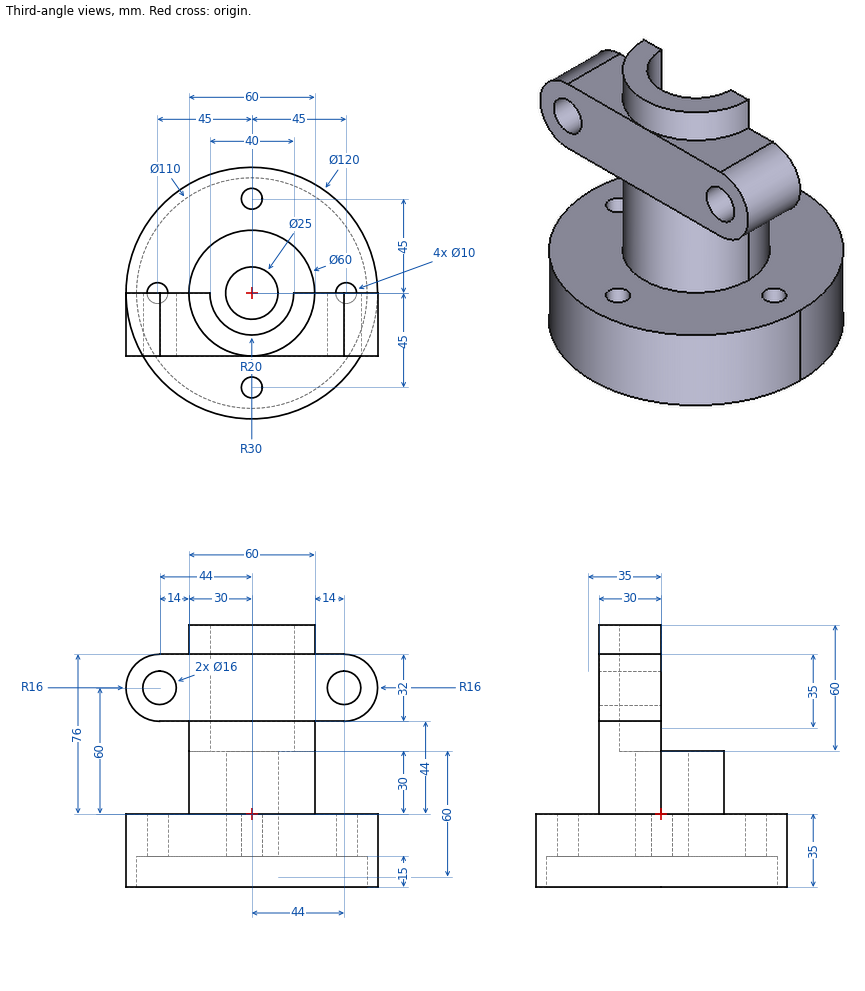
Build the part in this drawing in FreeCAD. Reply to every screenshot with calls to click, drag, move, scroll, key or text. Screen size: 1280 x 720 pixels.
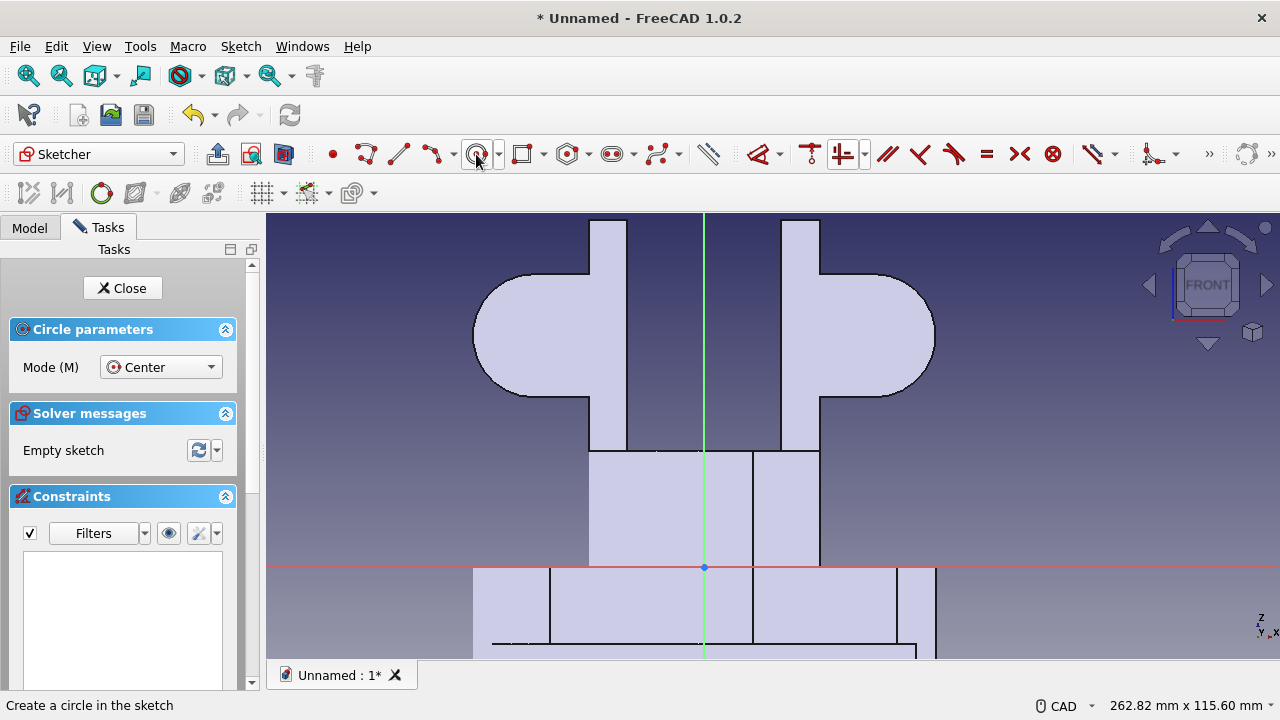
click(535, 336)
move(556, 314)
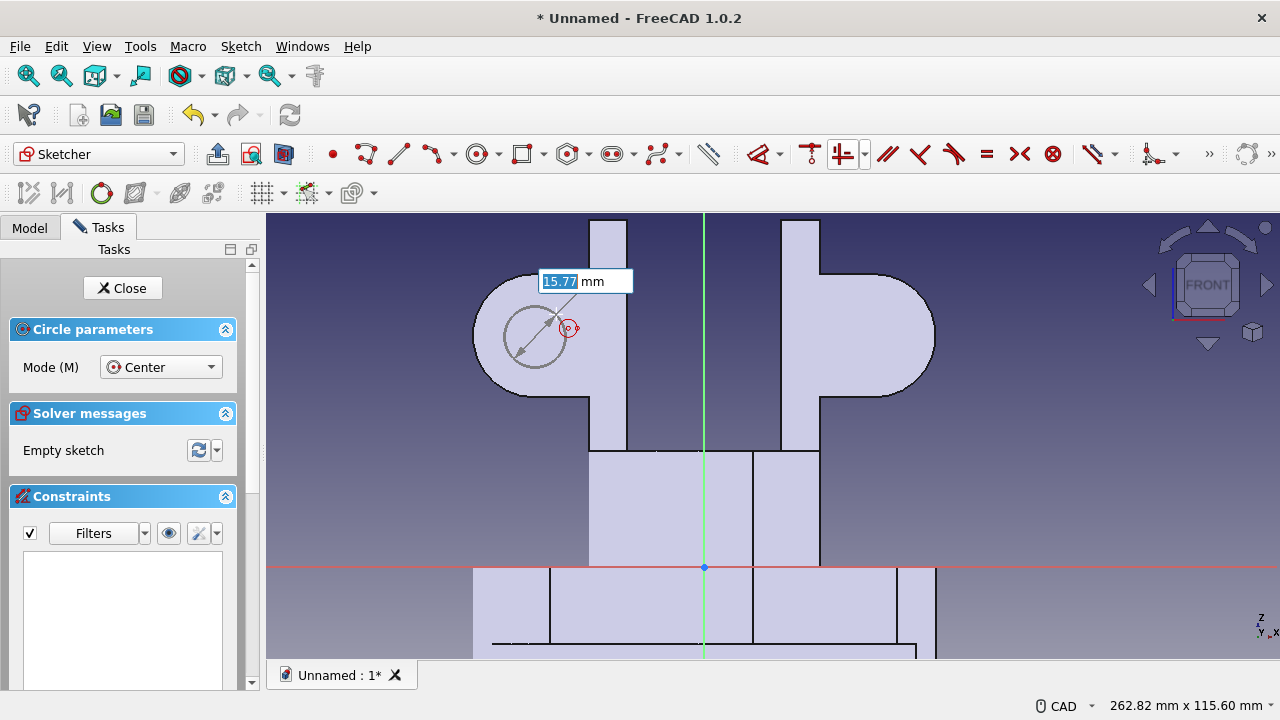
text(16)
key(Return)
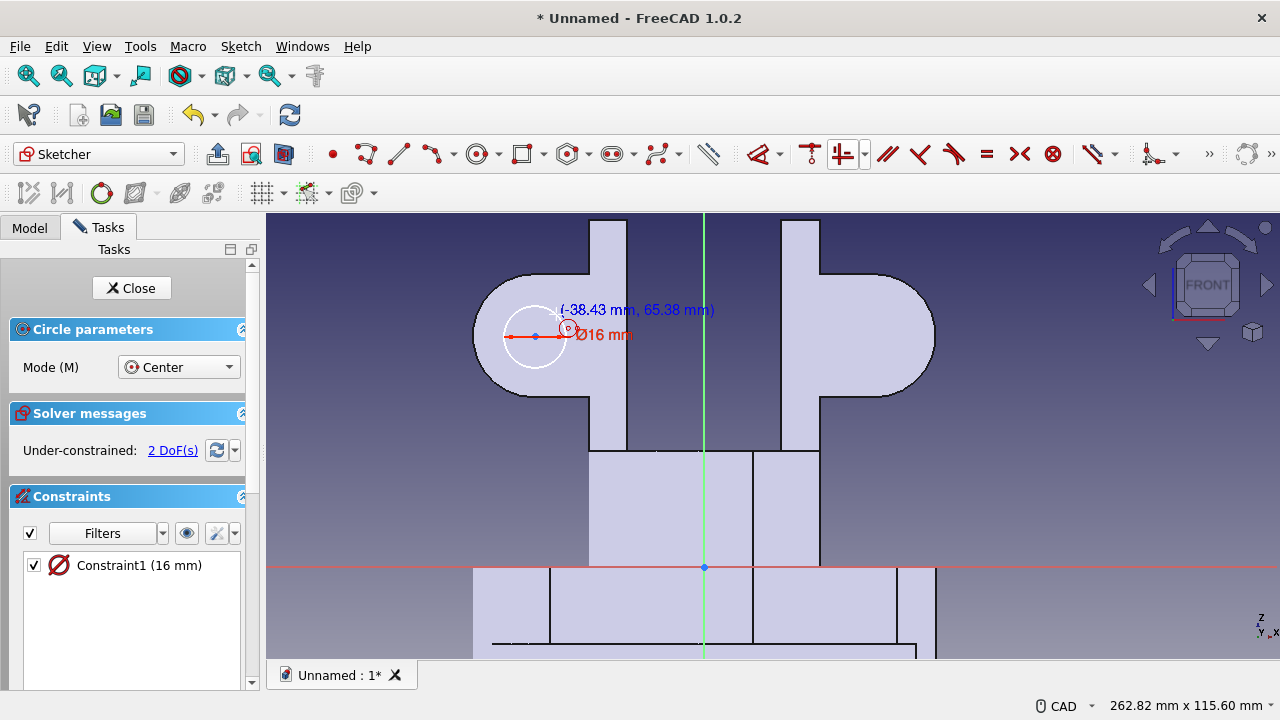
click(874, 336)
move(896, 314)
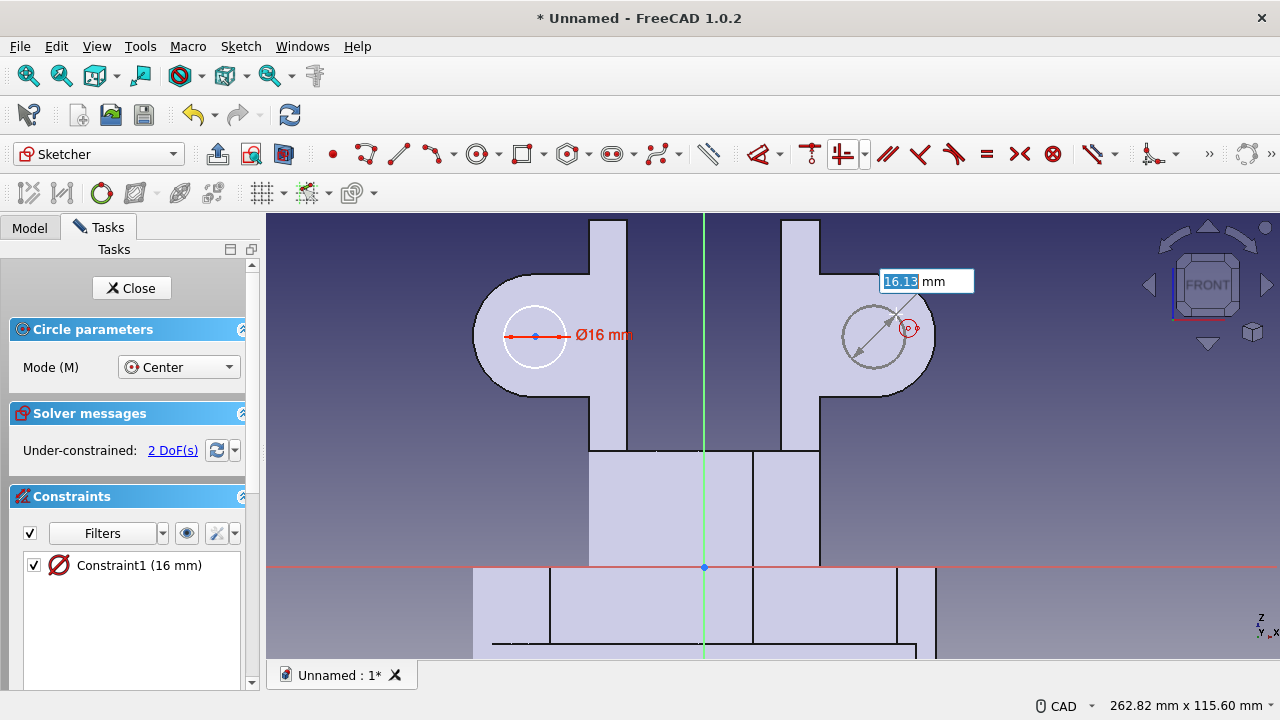
text(16)
key(Return)
key(Escape)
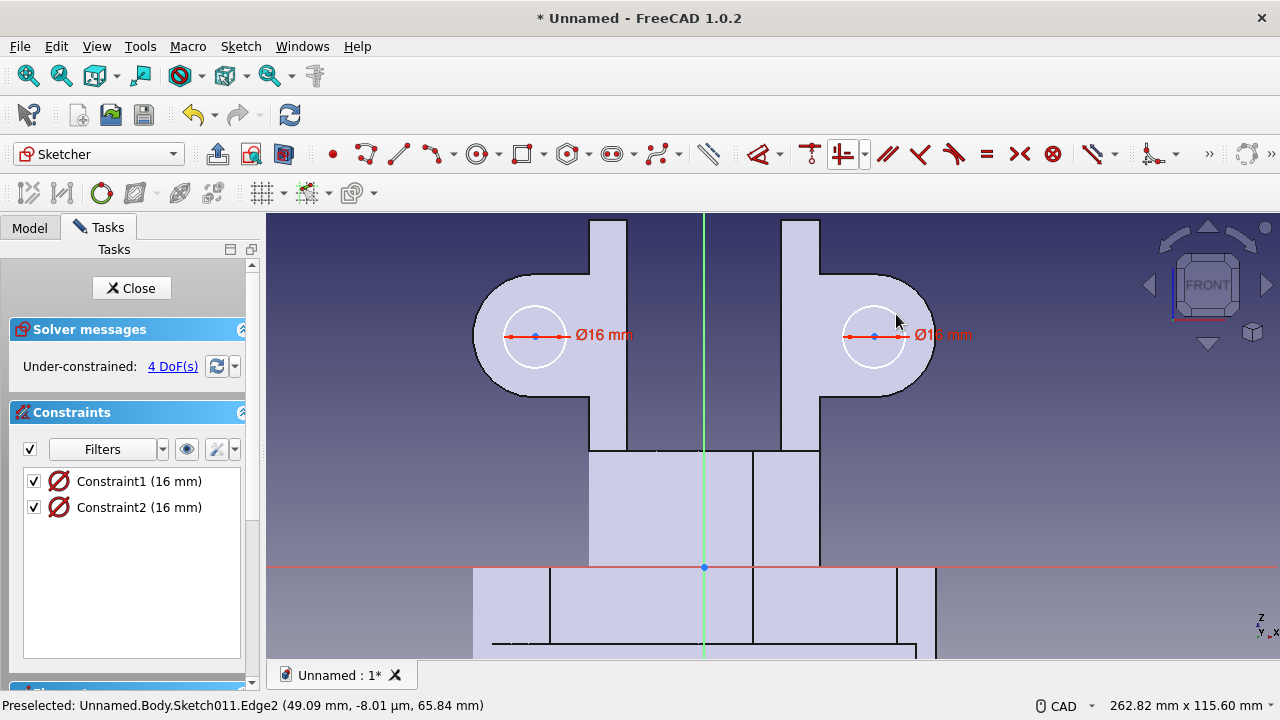
click(535, 337)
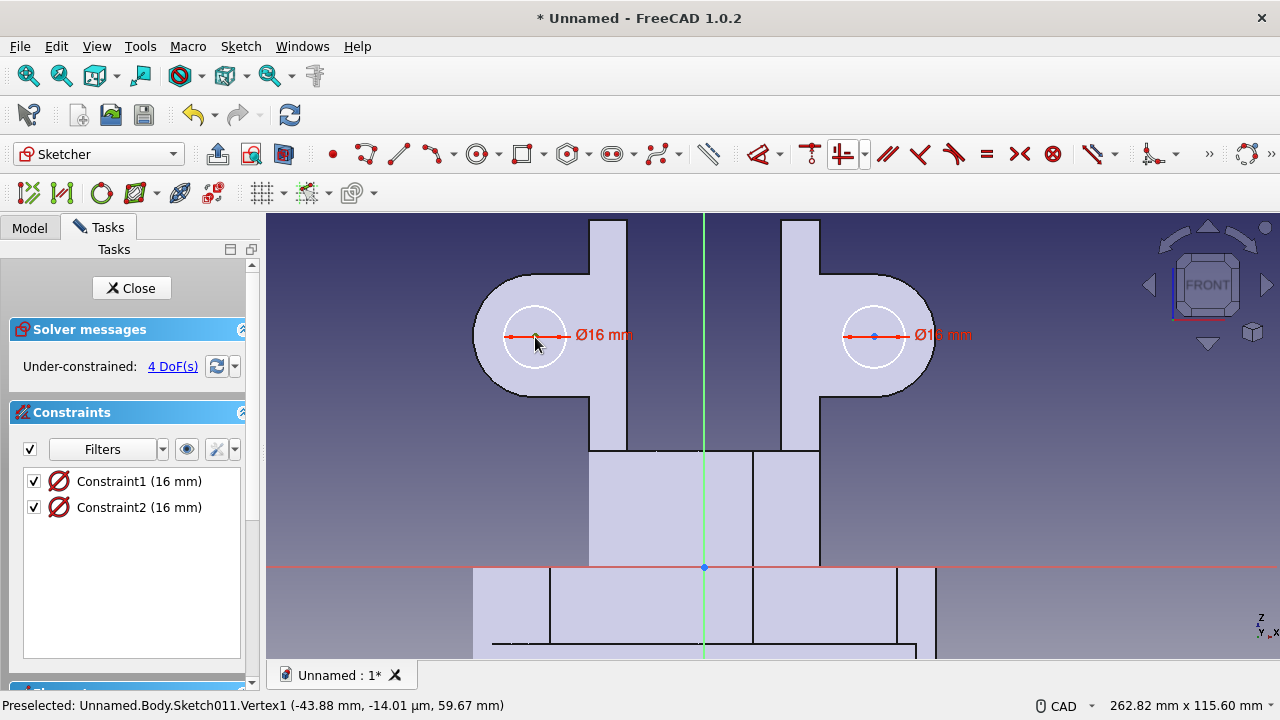
click(874, 337)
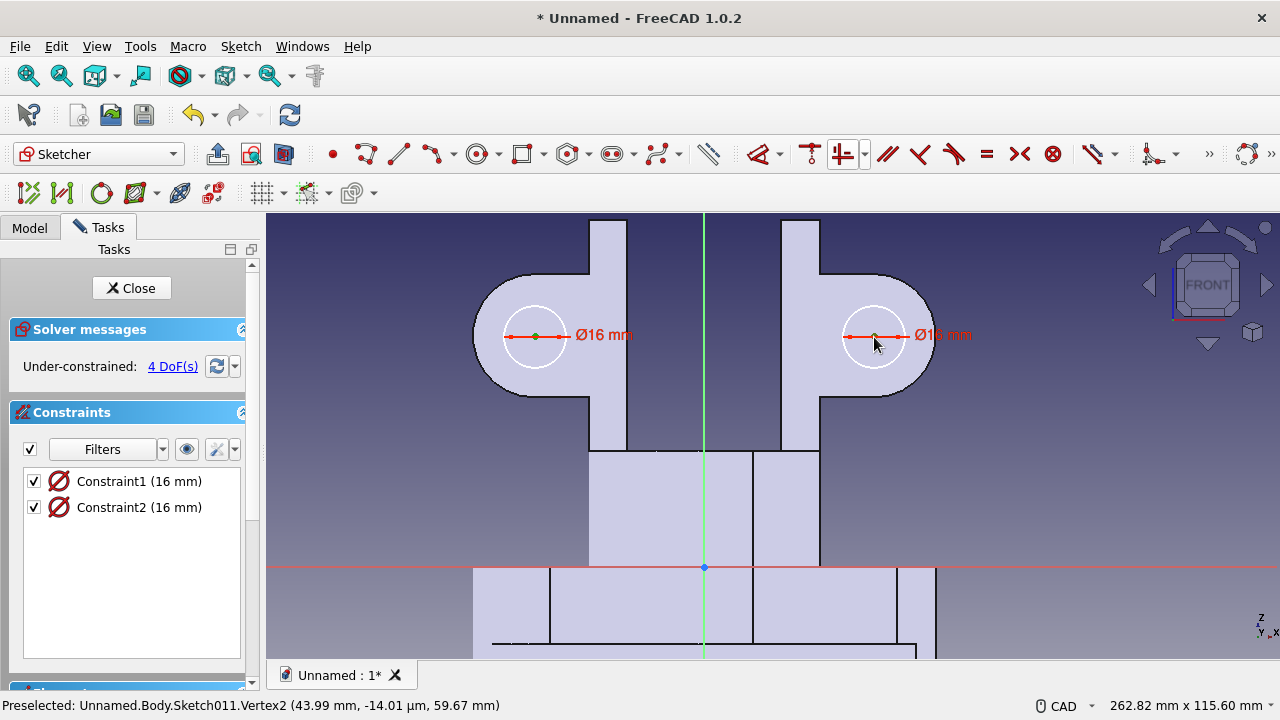
click(864, 154)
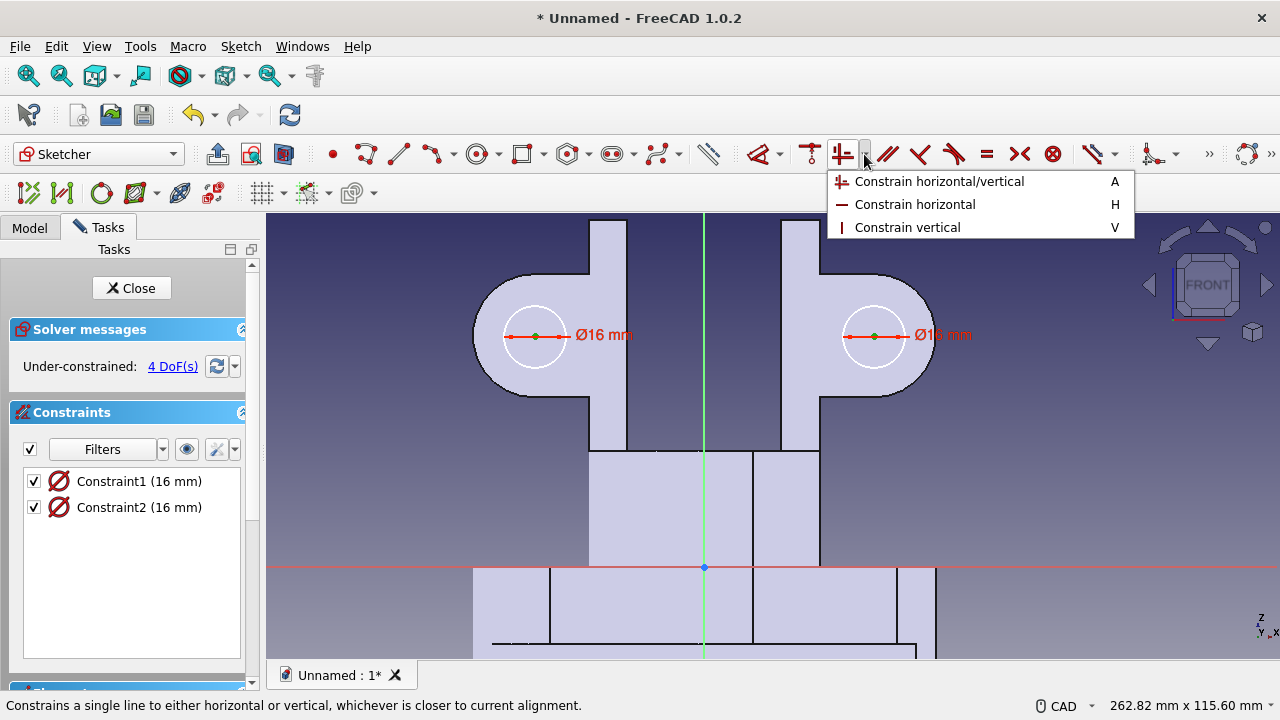
click(981, 204)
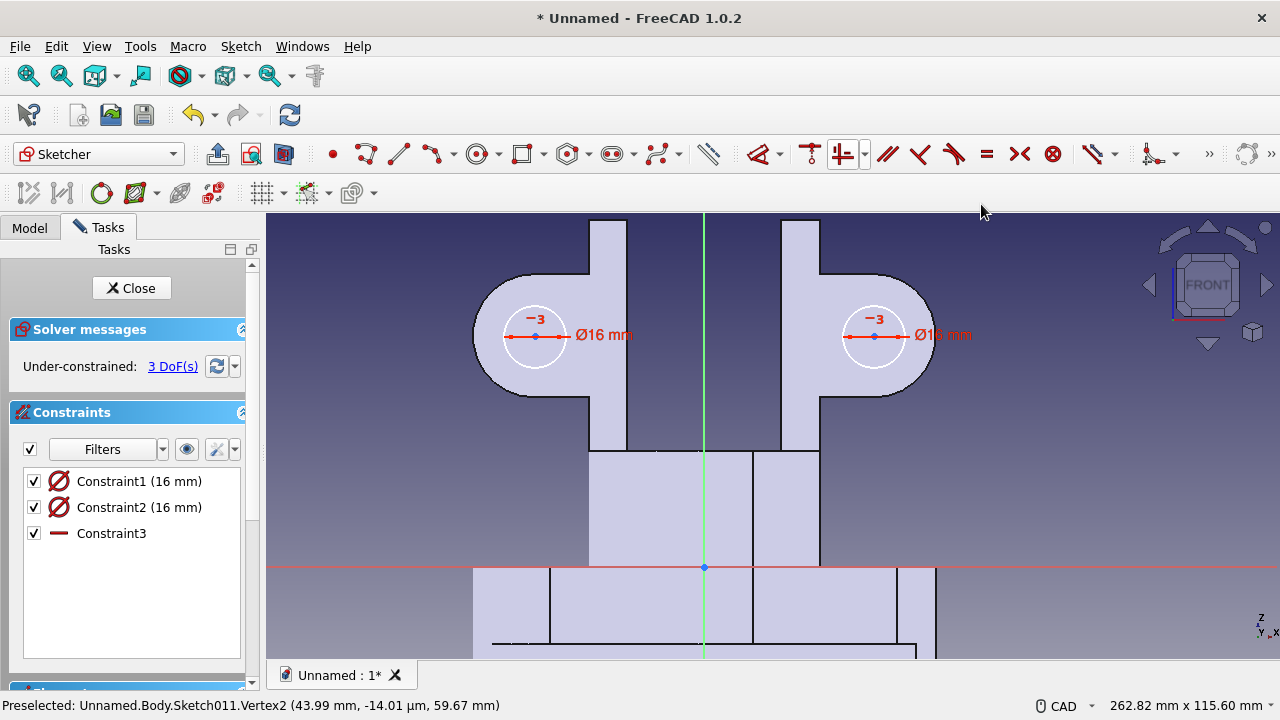
click(758, 154)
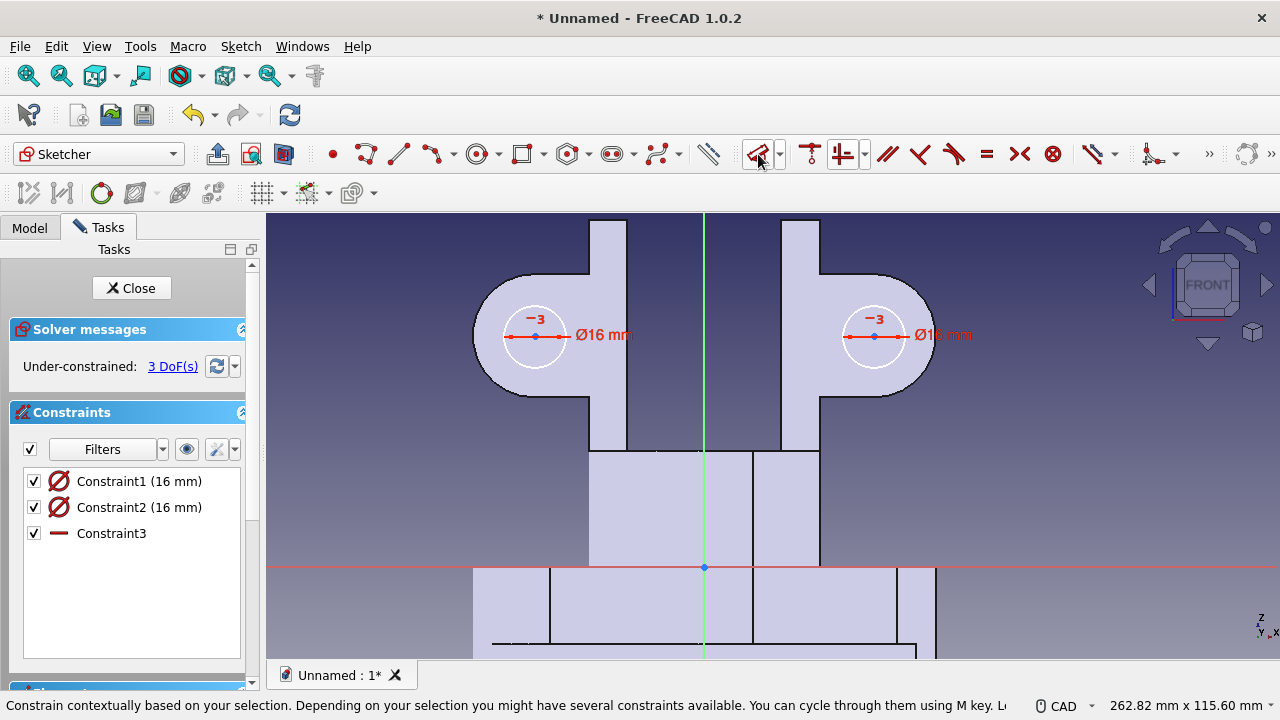
click(535, 337)
click(620, 601)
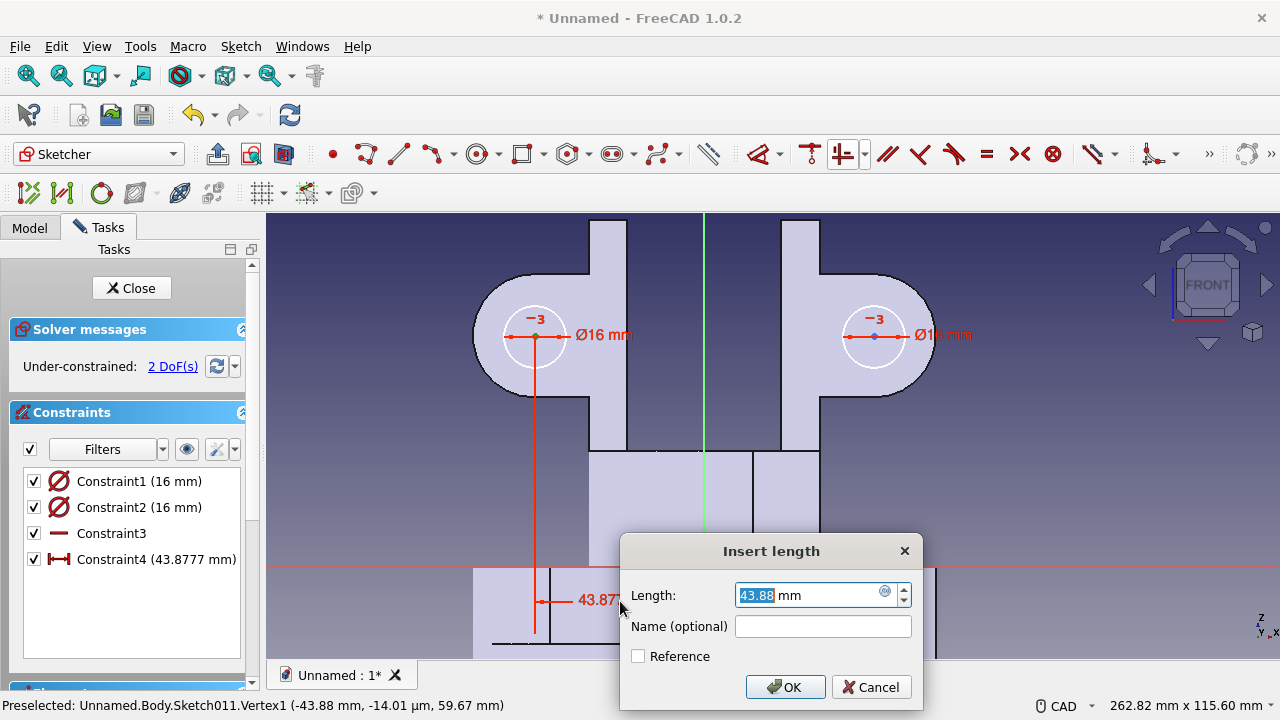
text(44)
key(Return)